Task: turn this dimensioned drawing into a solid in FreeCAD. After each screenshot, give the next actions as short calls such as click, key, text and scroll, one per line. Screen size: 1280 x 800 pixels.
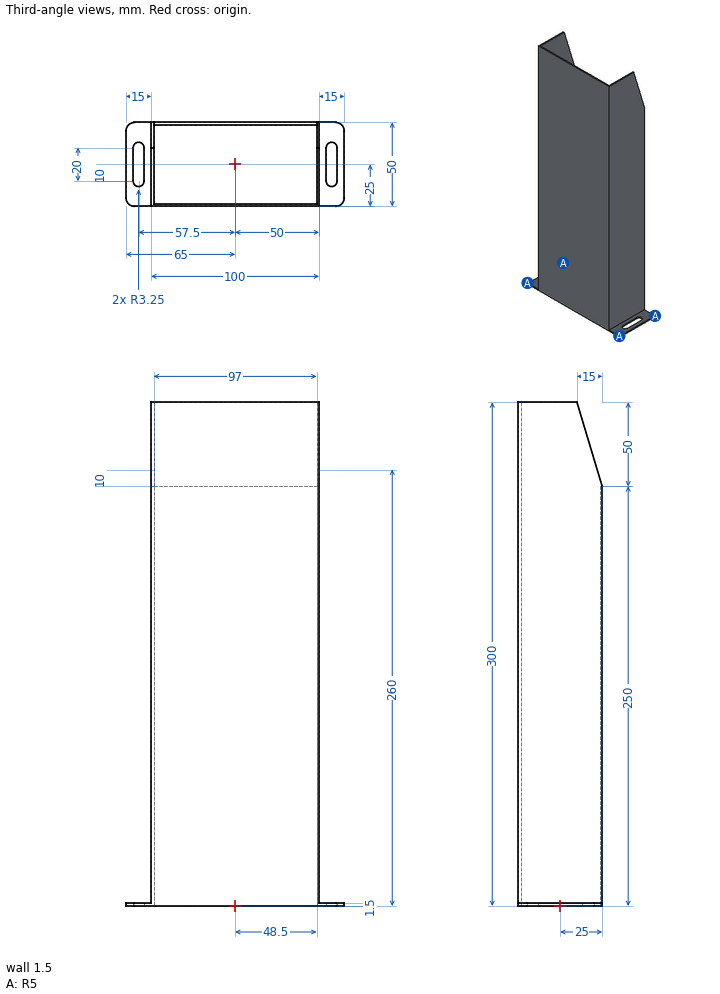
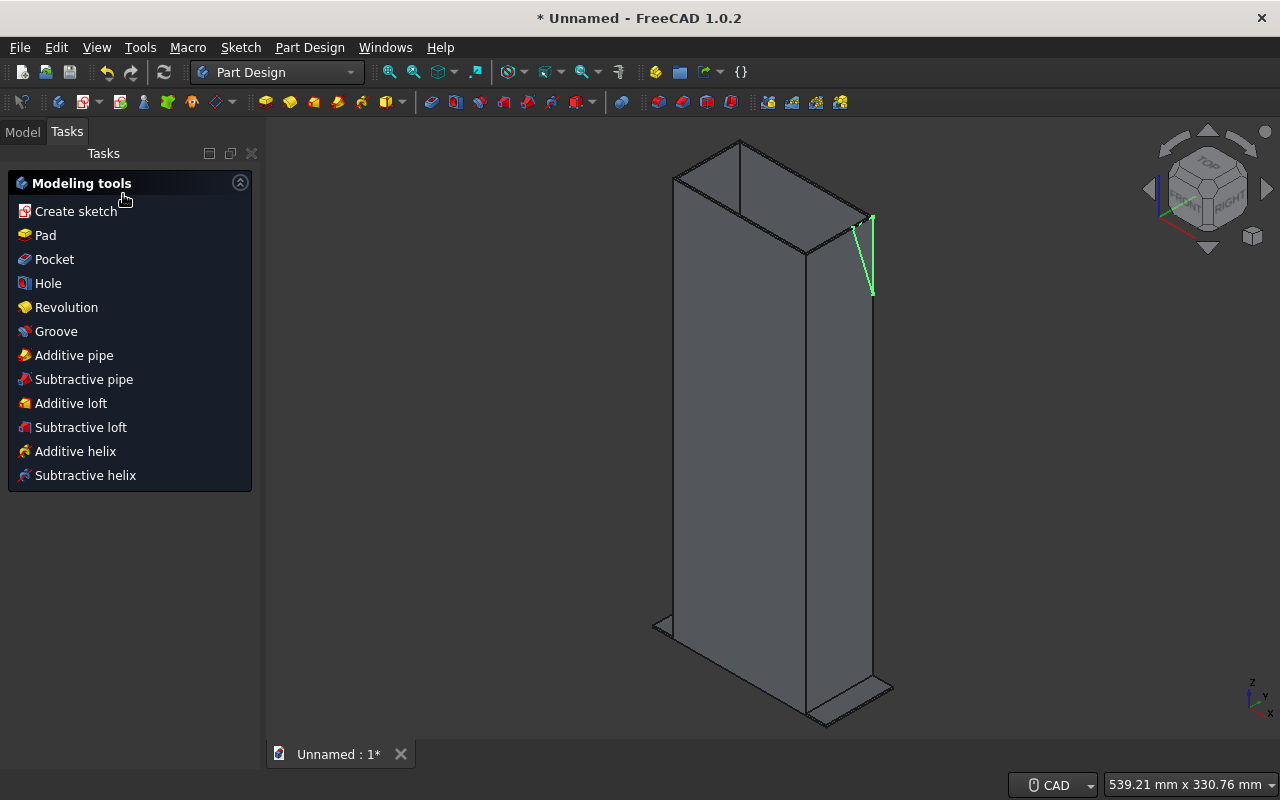
click(432, 102)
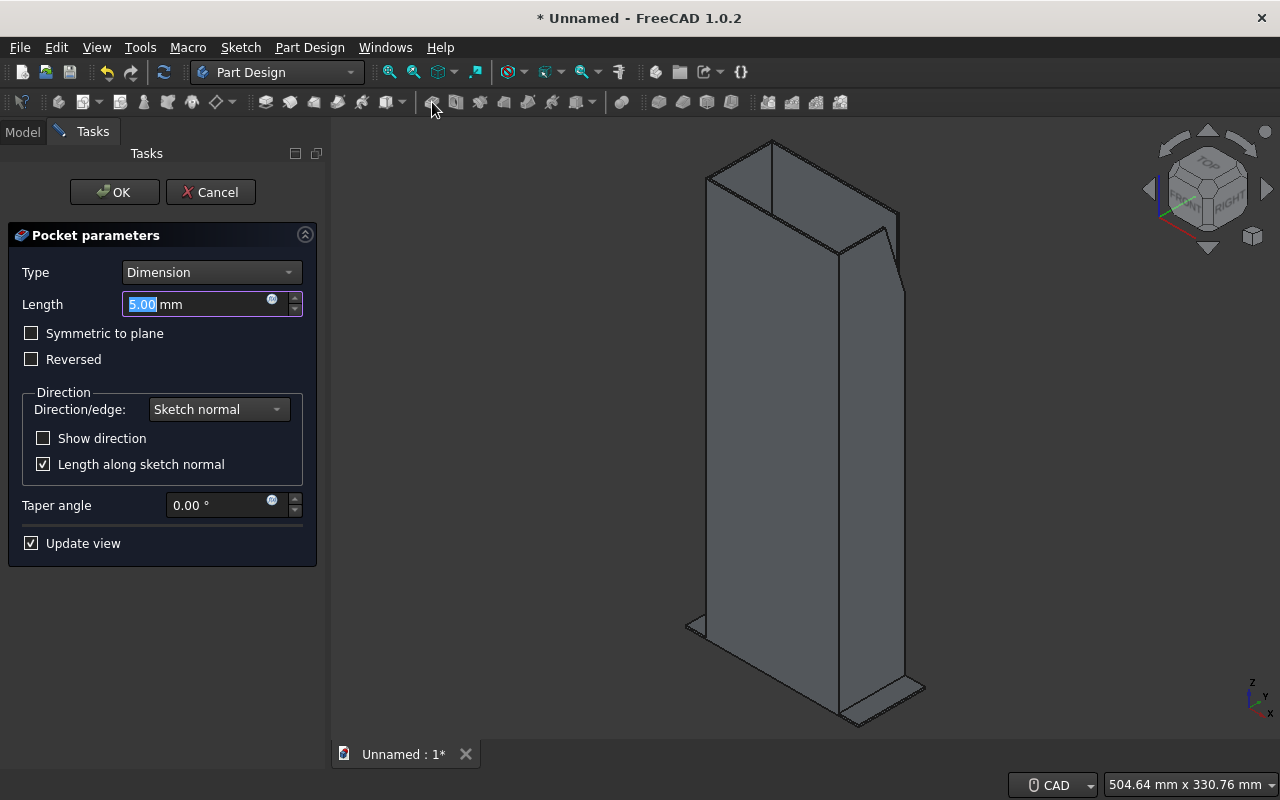
click(212, 272)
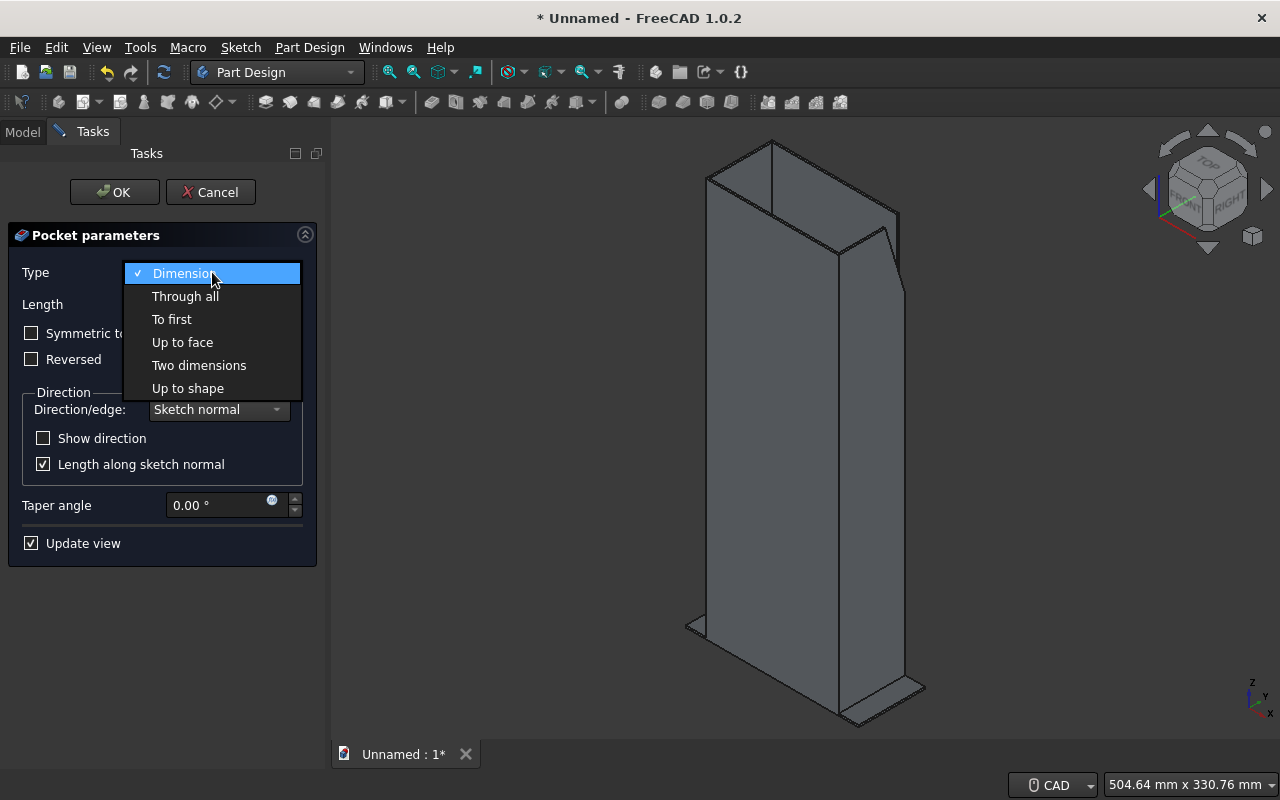
click(212, 296)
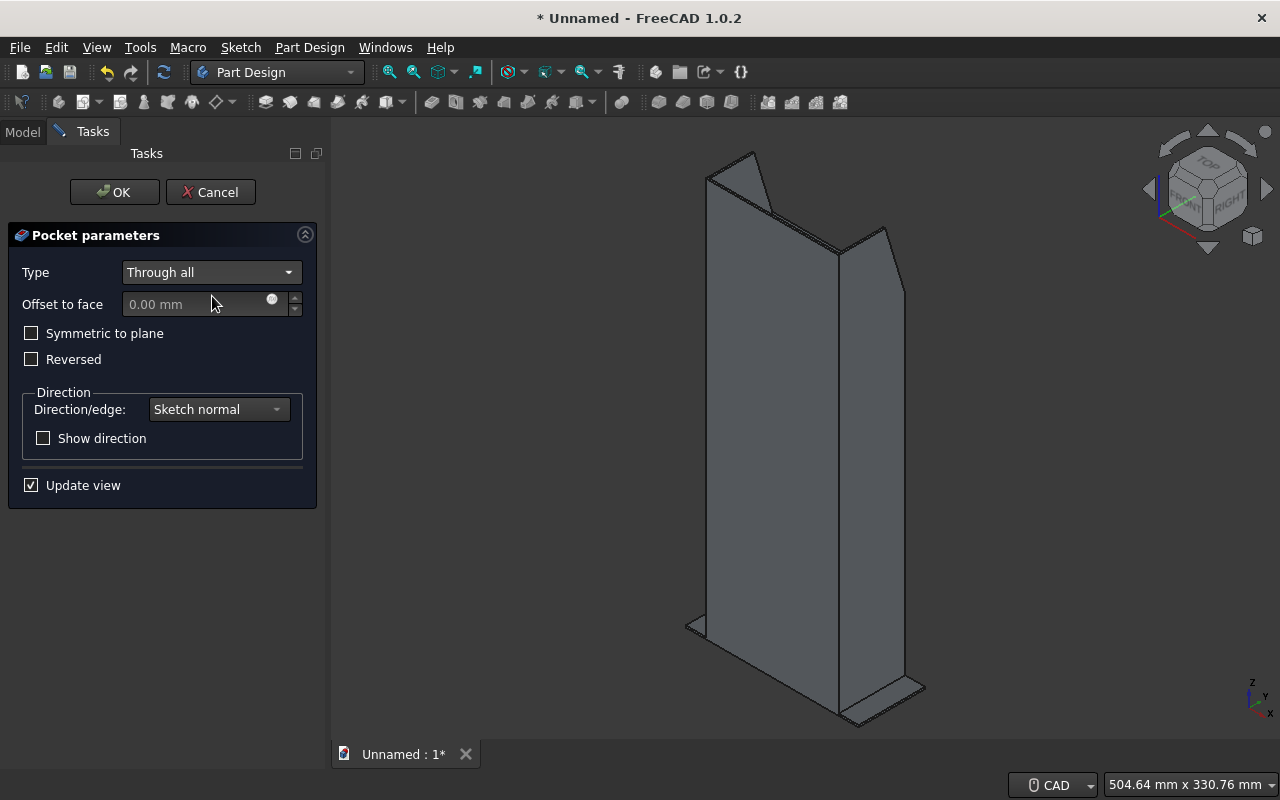
click(115, 192)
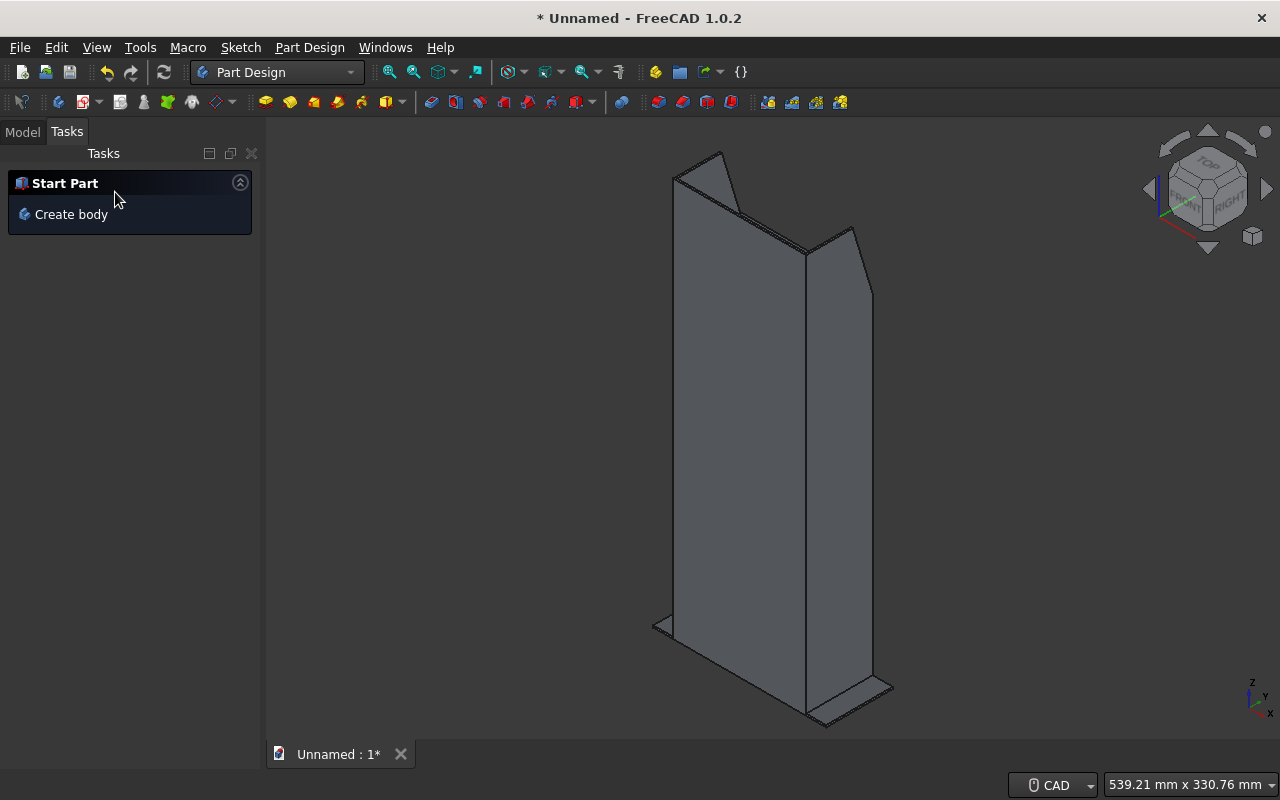
key(2)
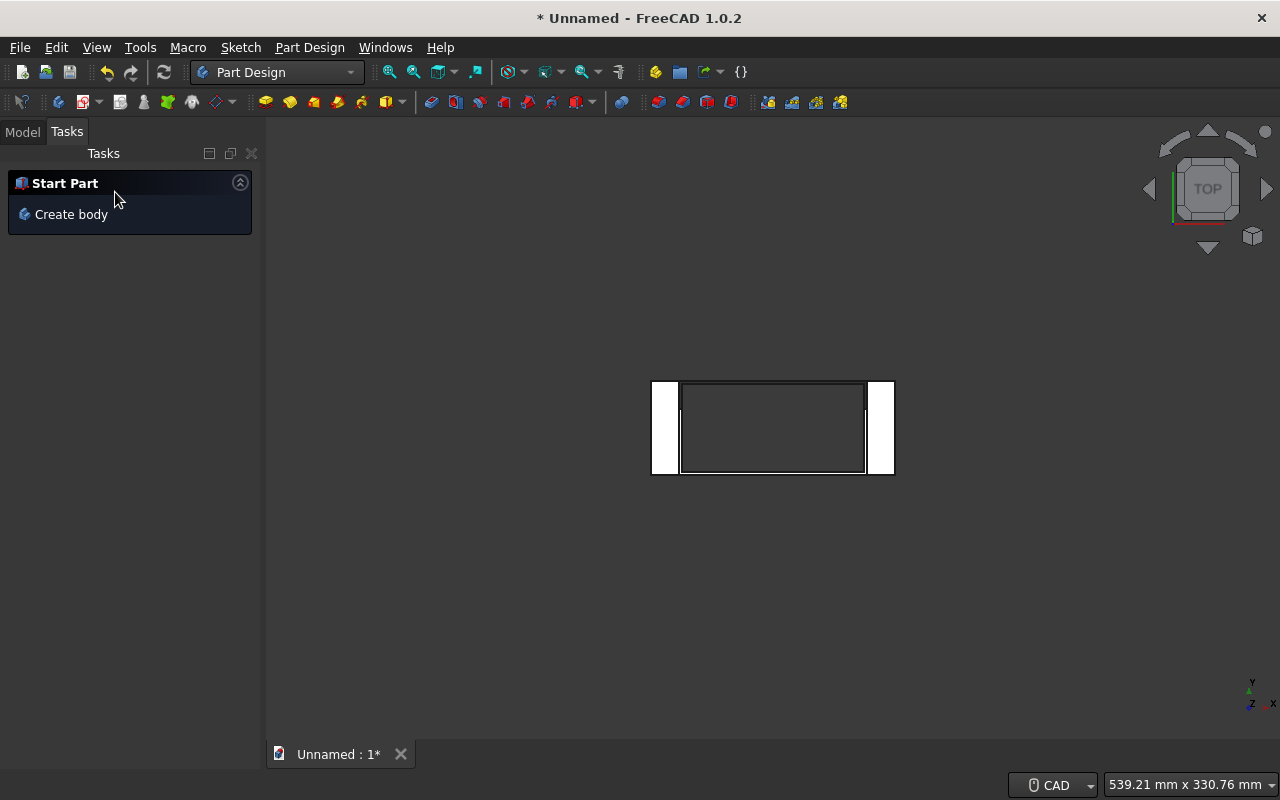
click(390, 72)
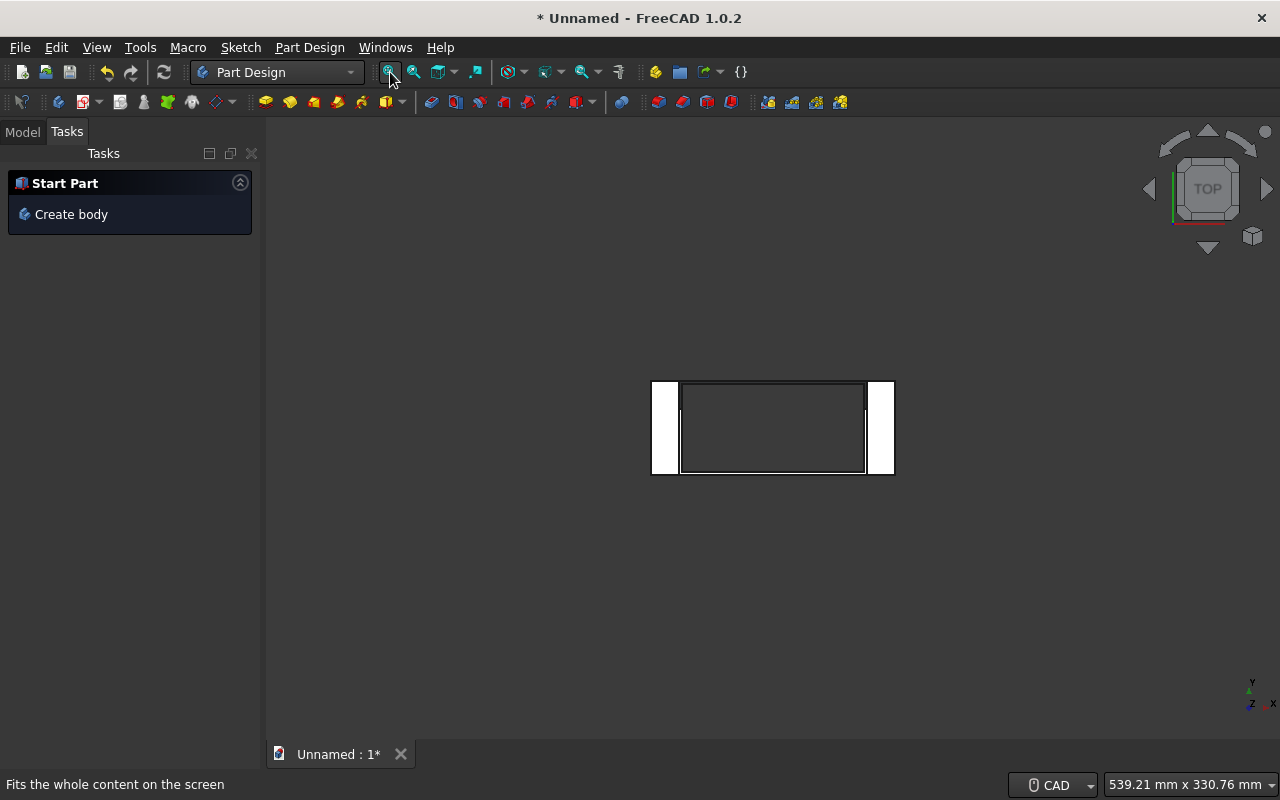
scroll(895, 474, up, 14)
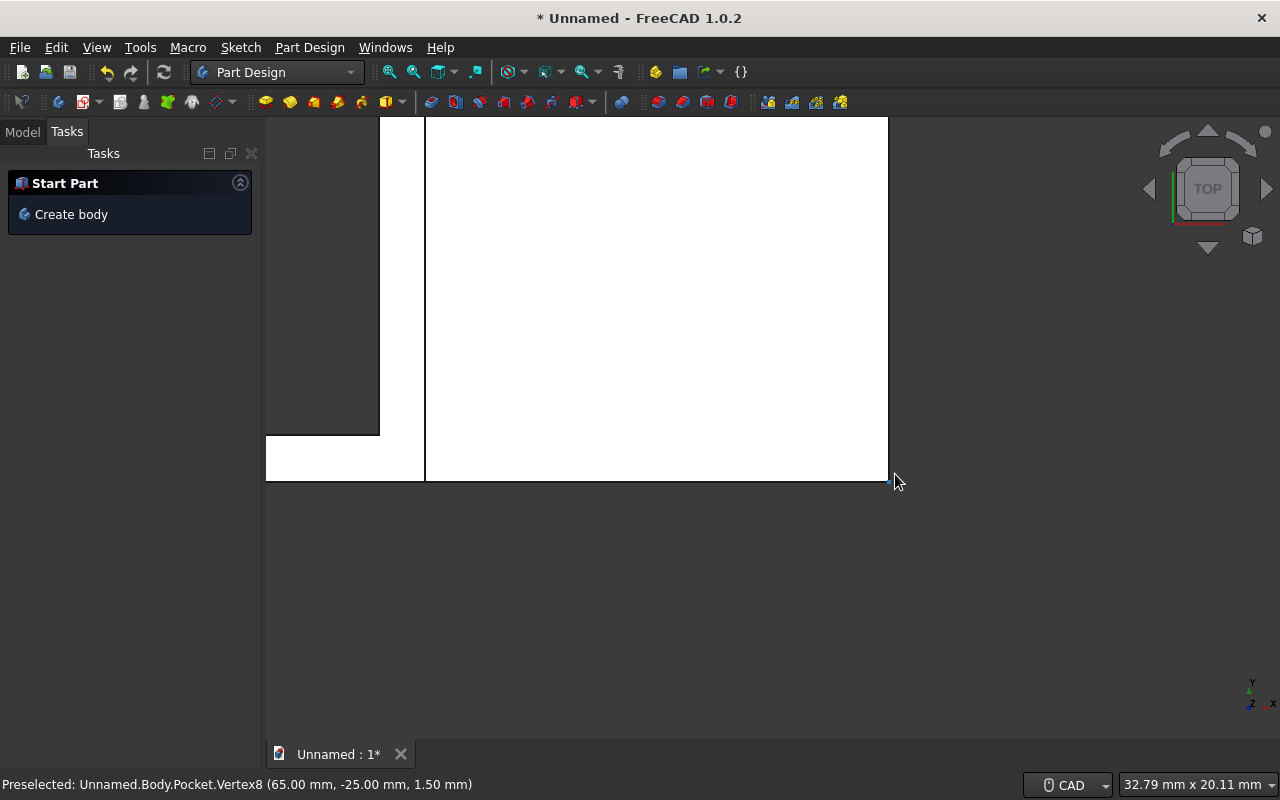
click(390, 72)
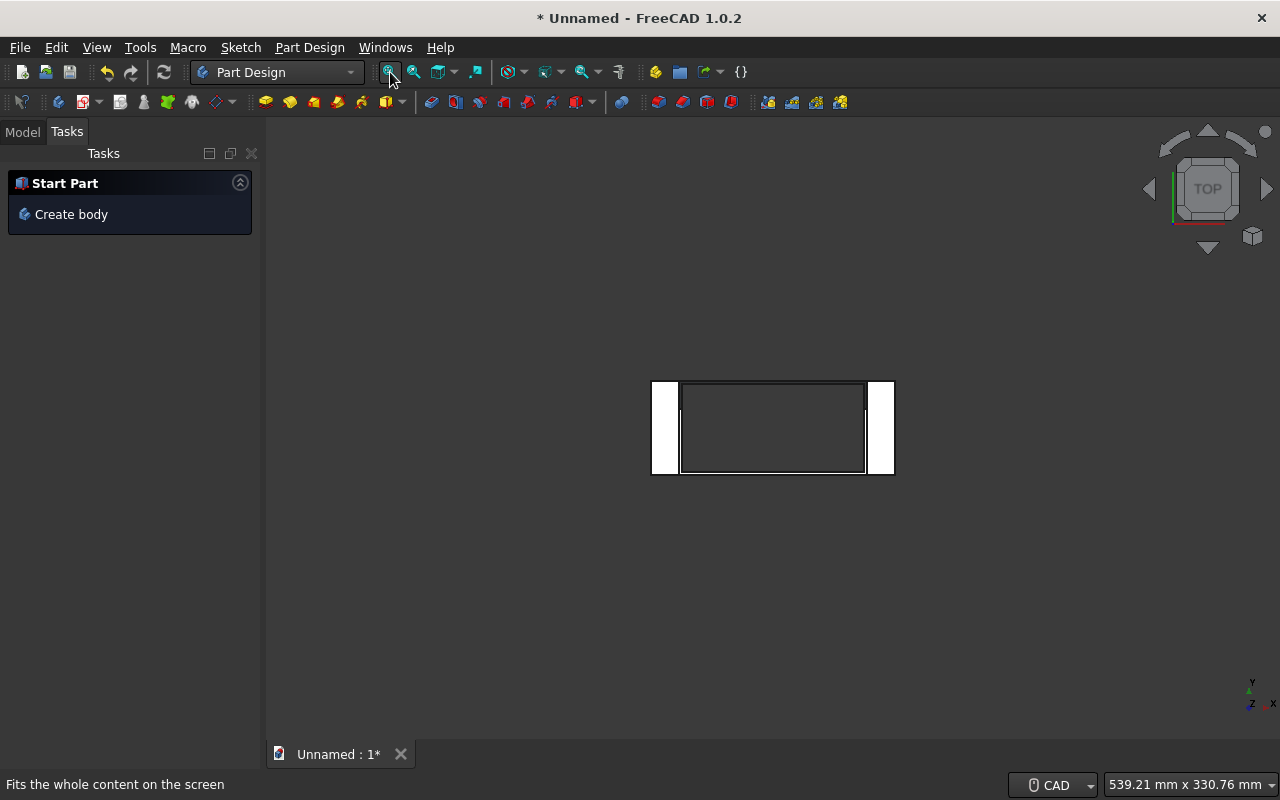
key(0)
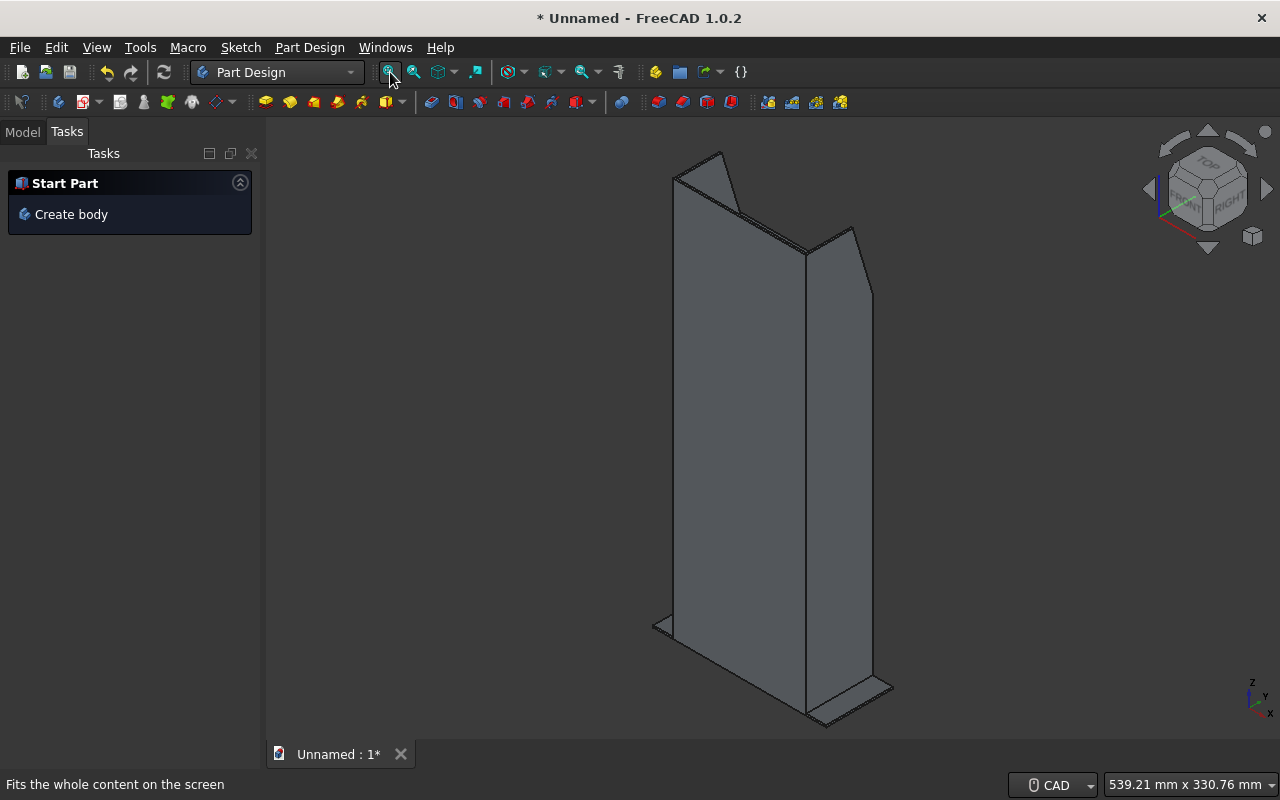
key(1)